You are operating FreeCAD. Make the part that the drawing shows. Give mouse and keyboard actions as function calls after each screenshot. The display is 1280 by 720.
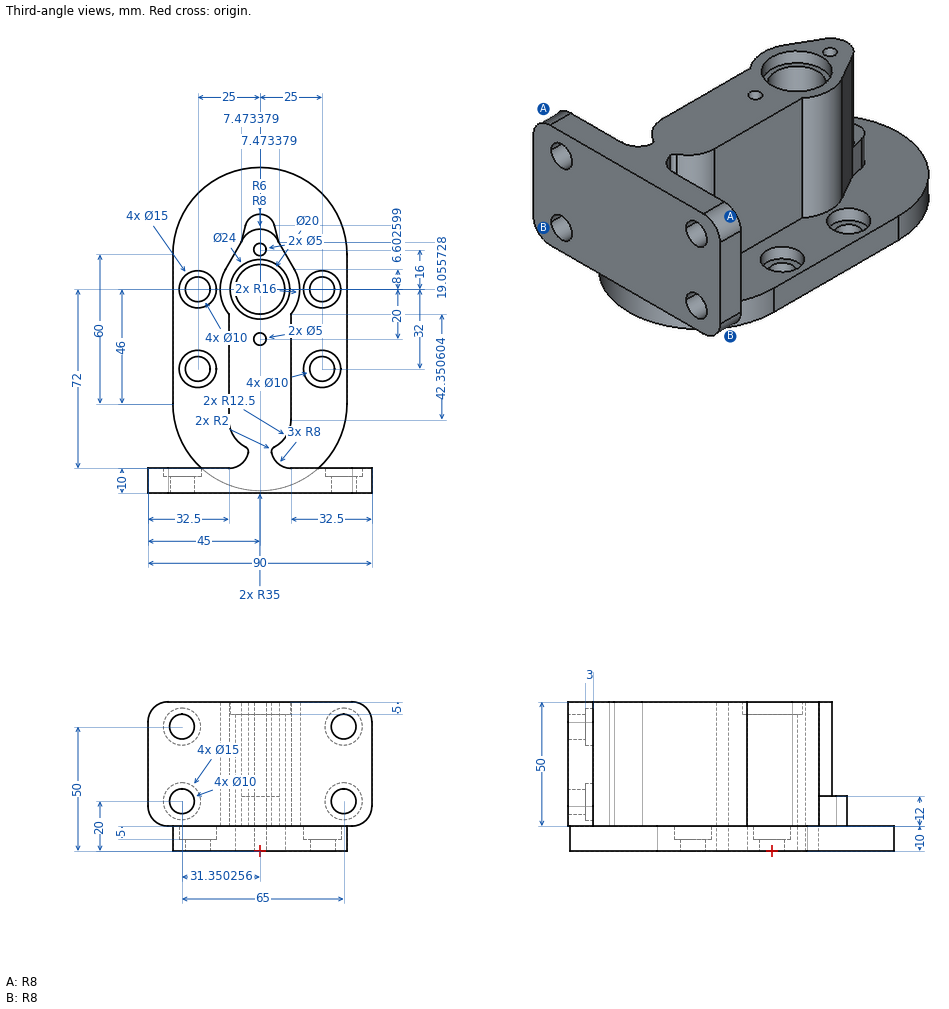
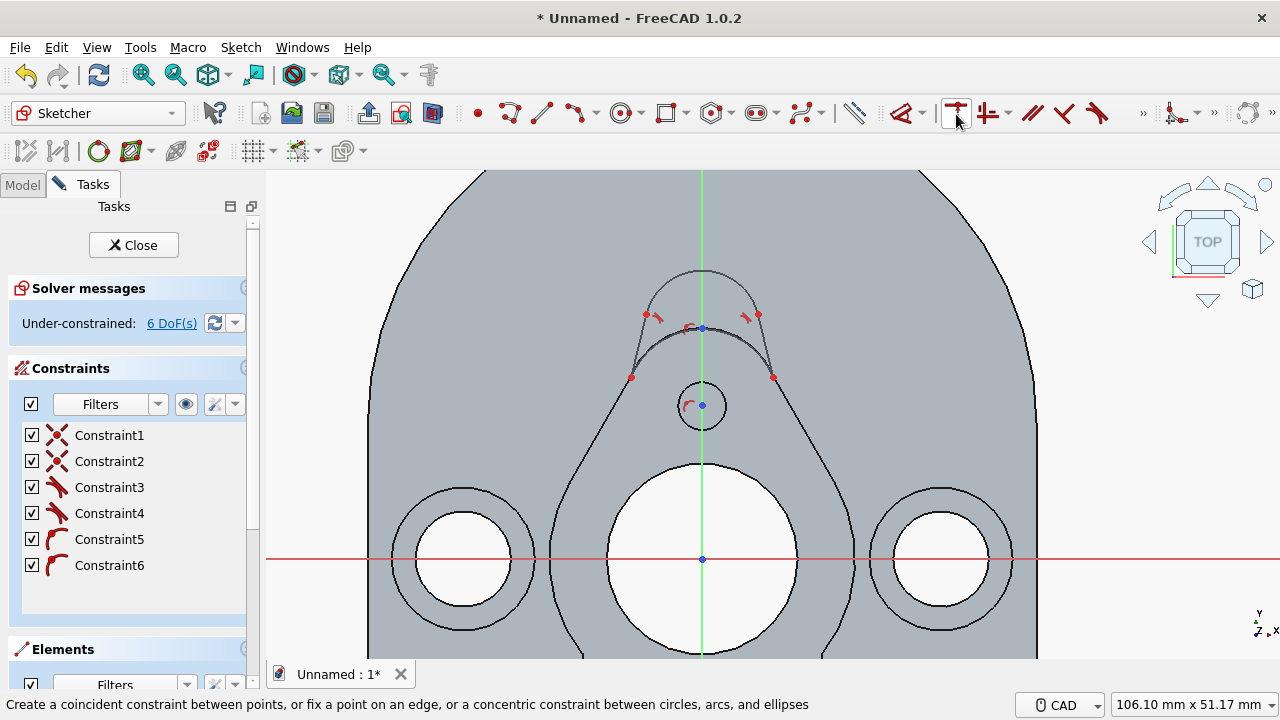
click(902, 114)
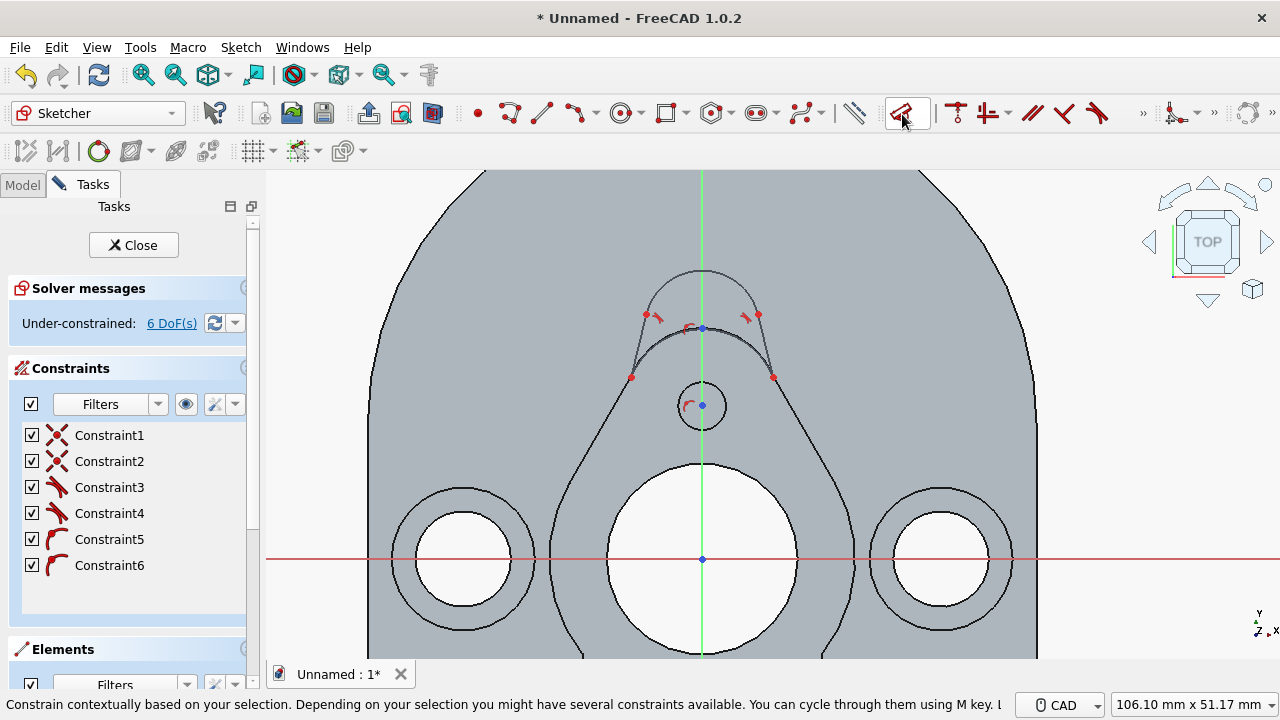
click(731, 279)
click(747, 251)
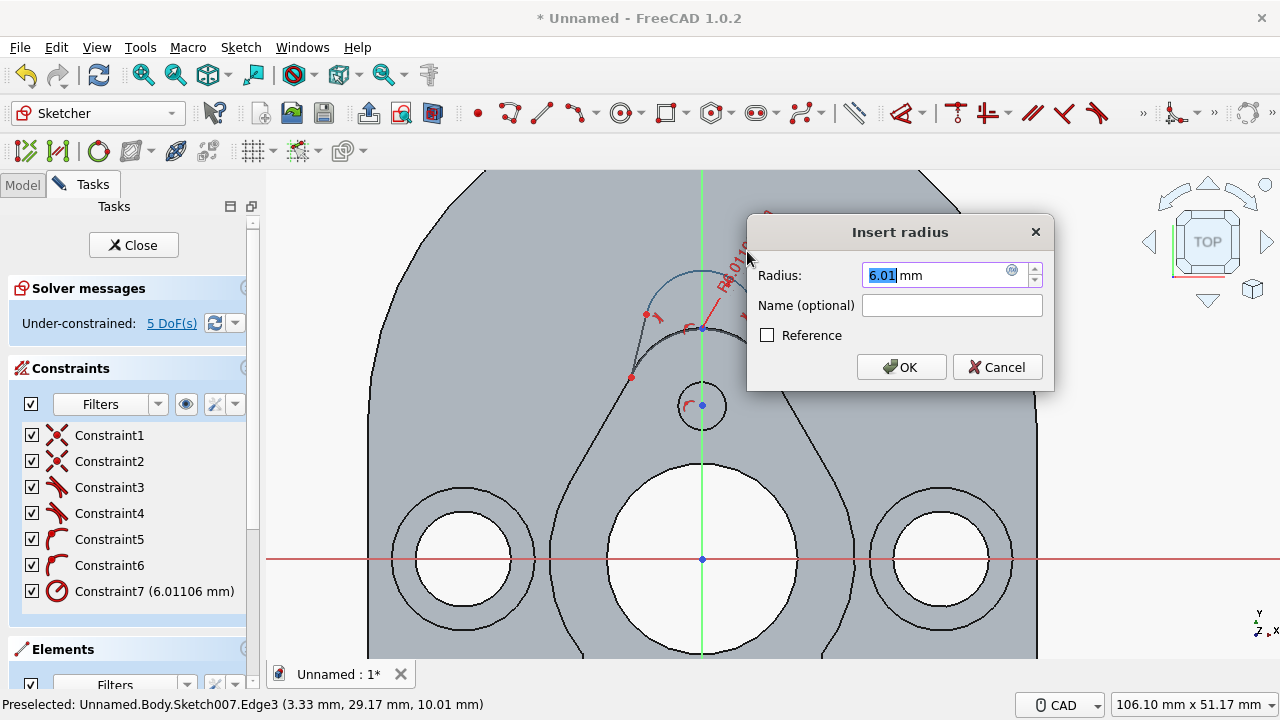
text(6)
key(Return)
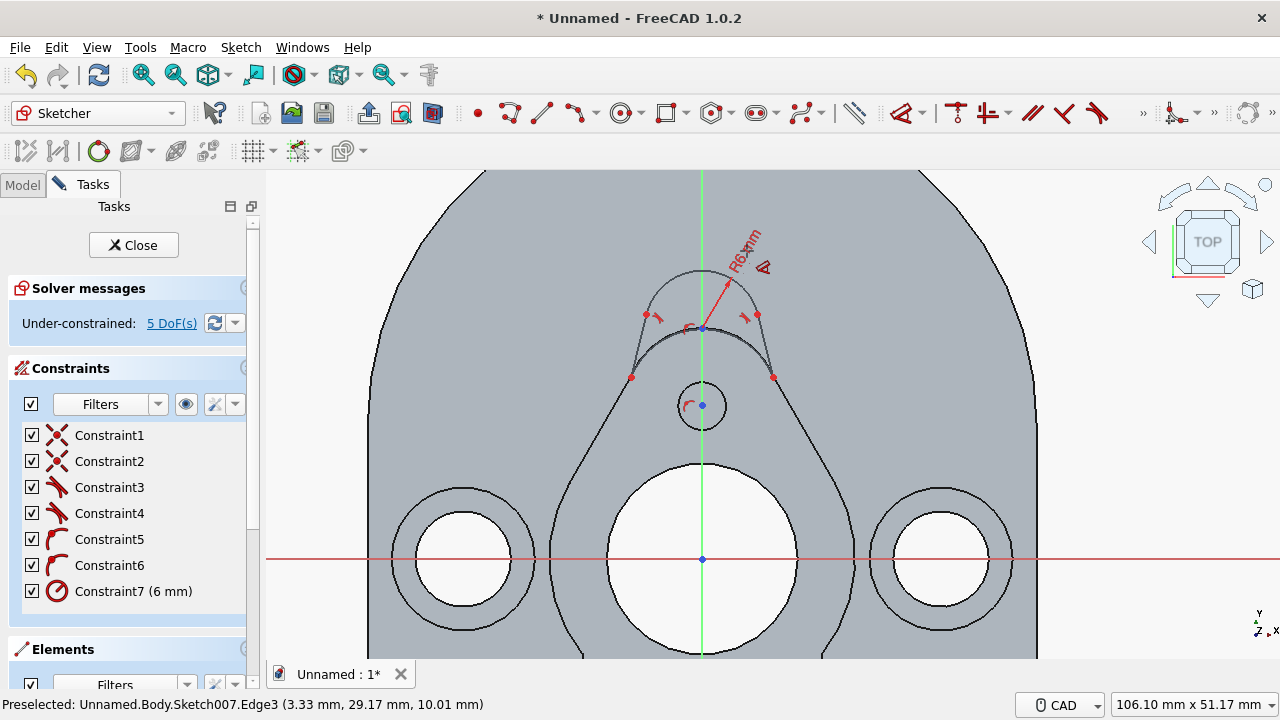
click(737, 338)
click(792, 345)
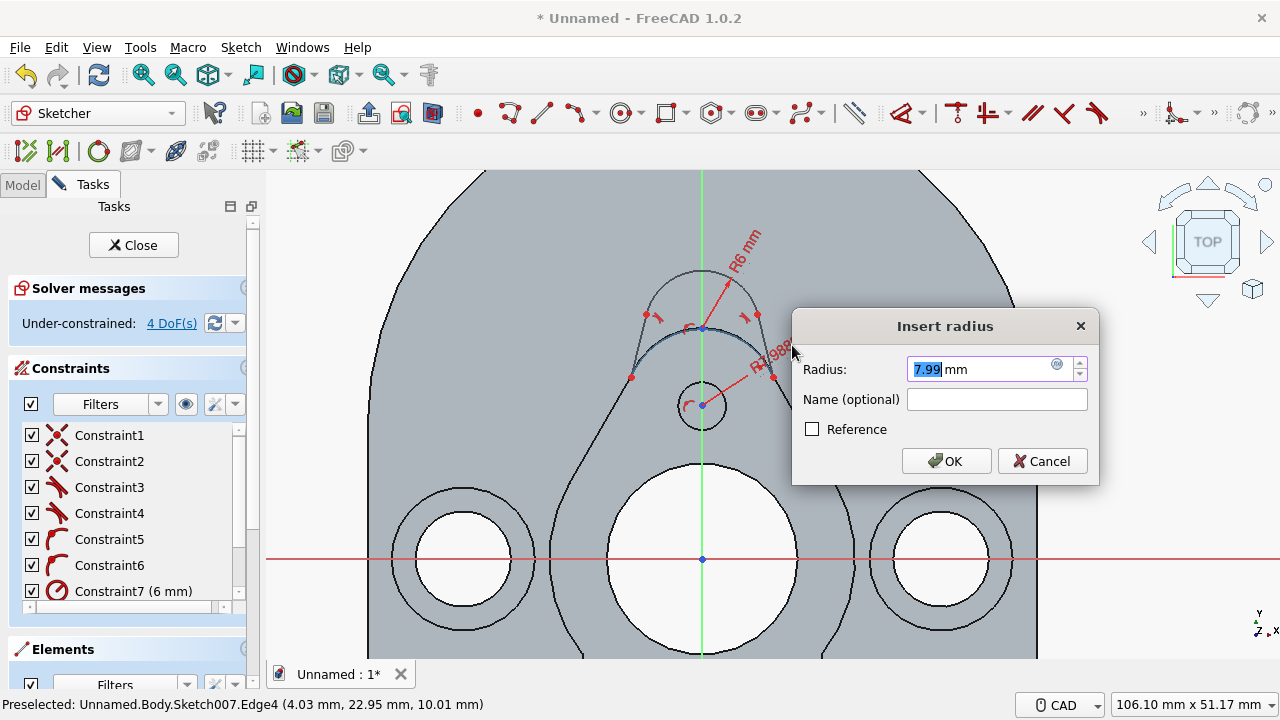
text(8)
key(Return)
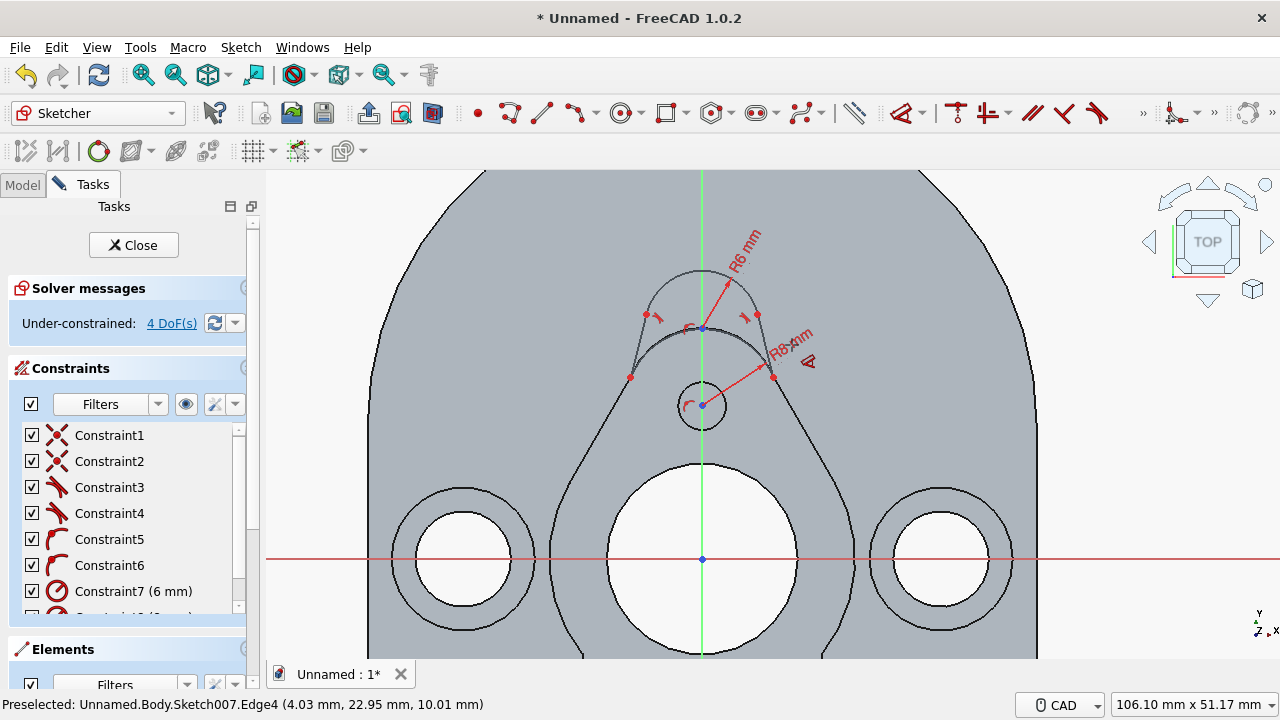
click(773, 378)
click(738, 593)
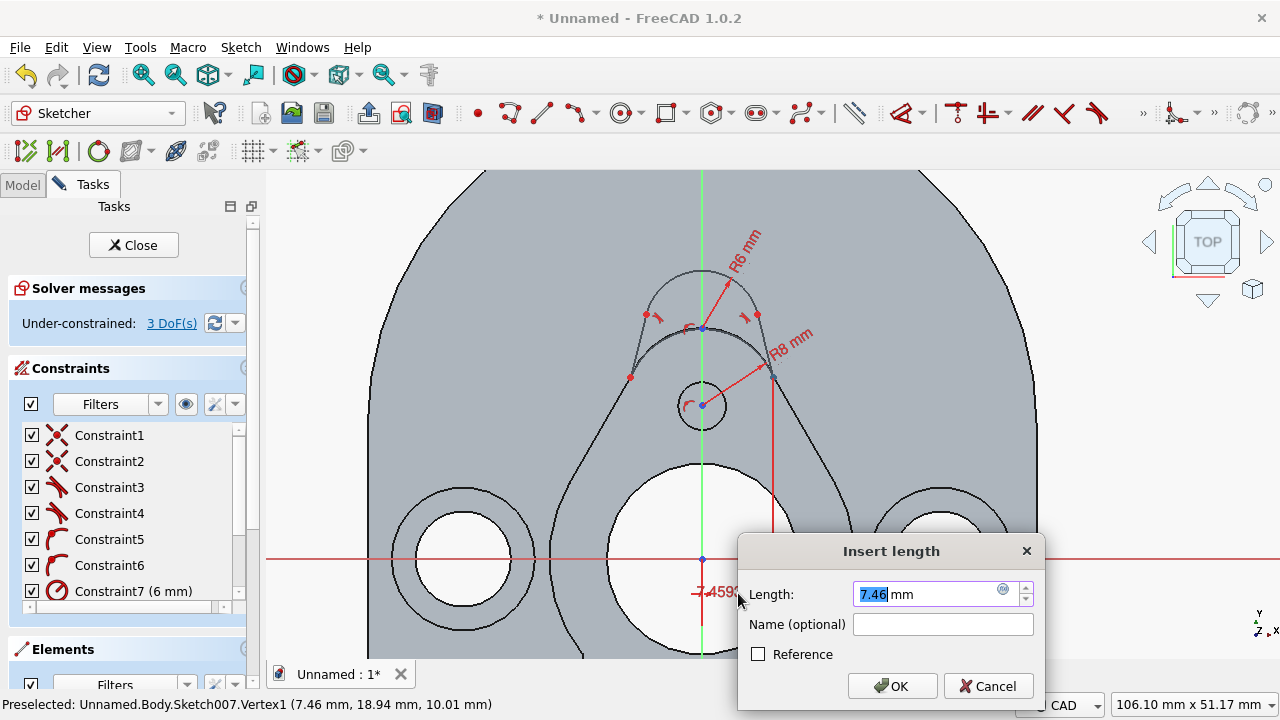
text(7.473379)
key(Return)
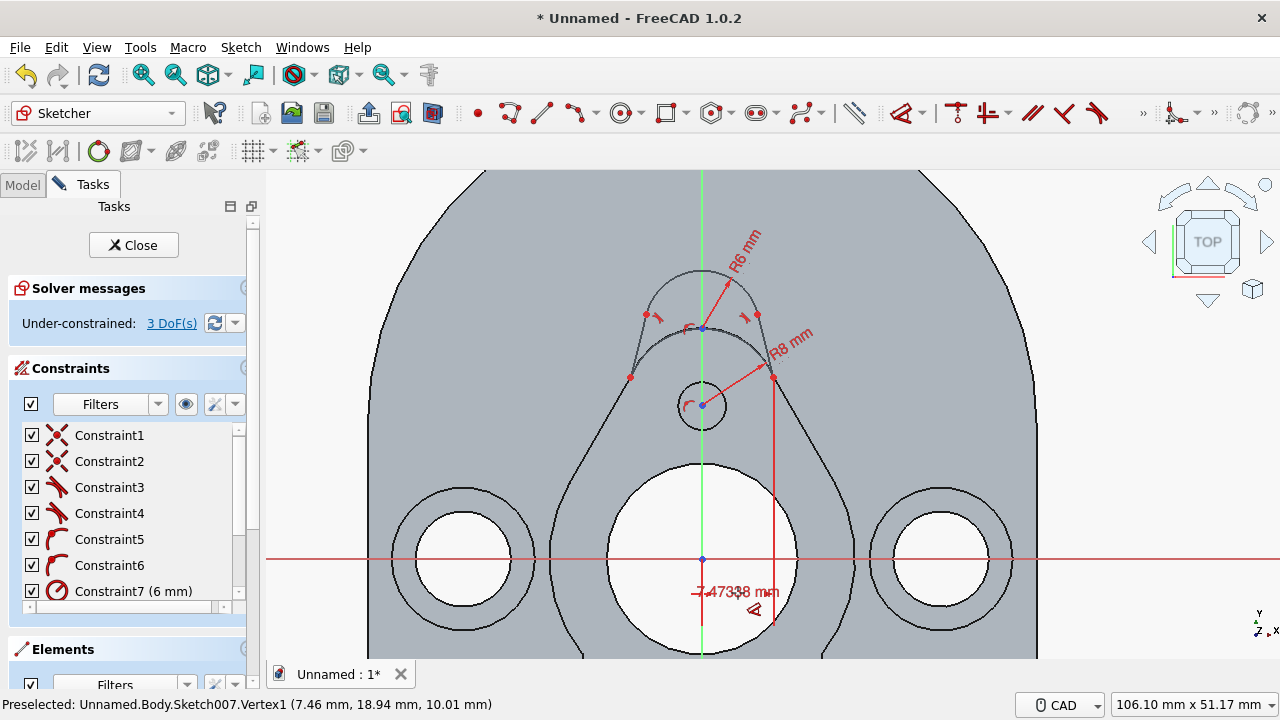
click(631, 378)
click(666, 593)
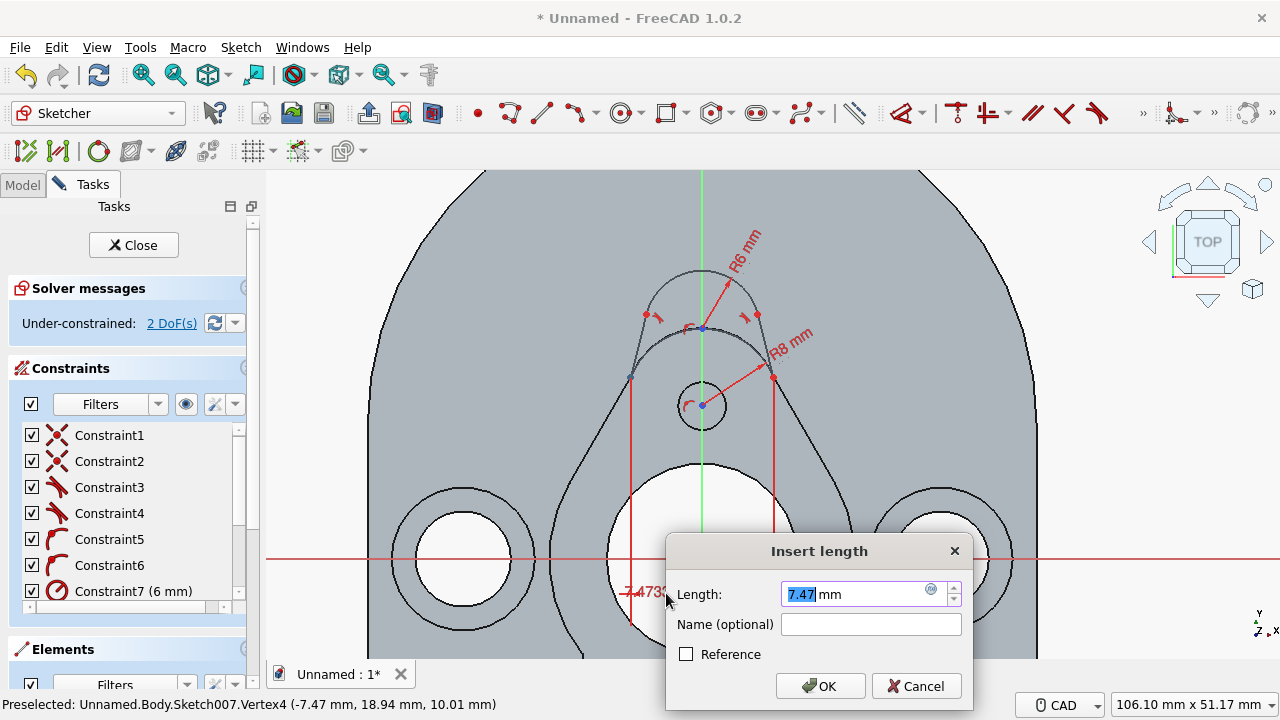
text(7.473379)
key(Return)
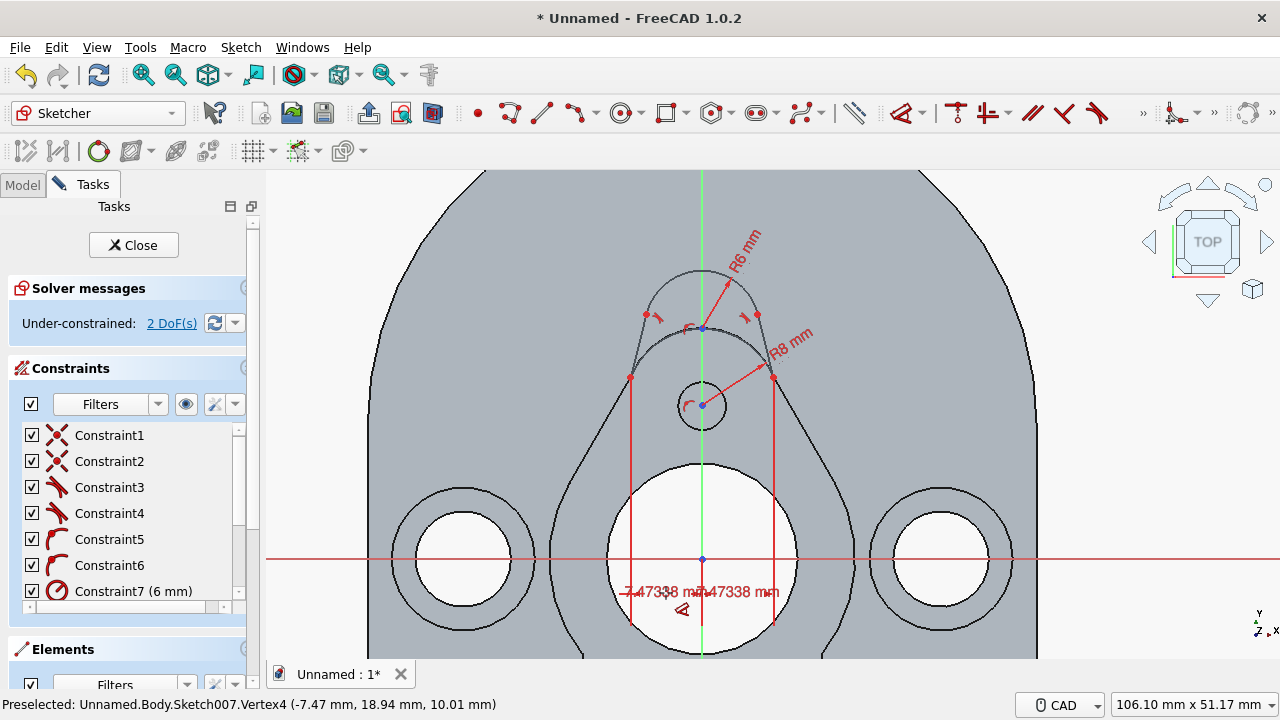
click(763, 333)
click(808, 324)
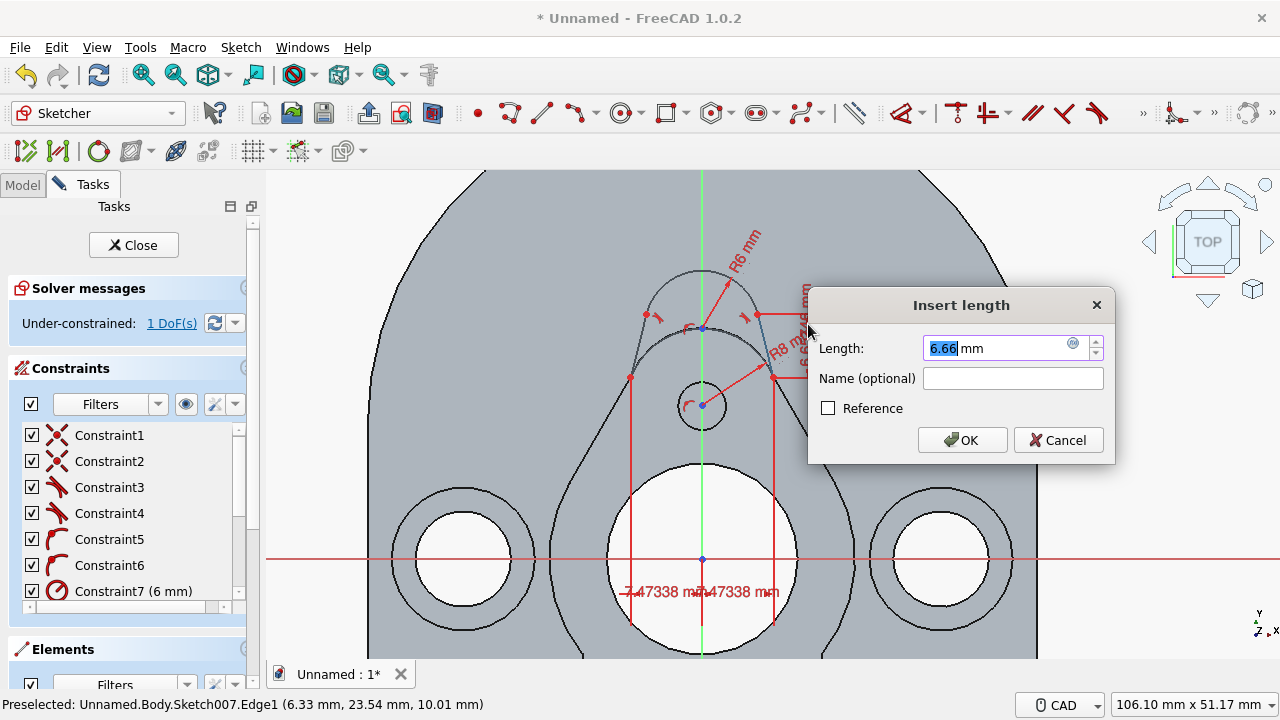
text(6.602599)
key(Return)